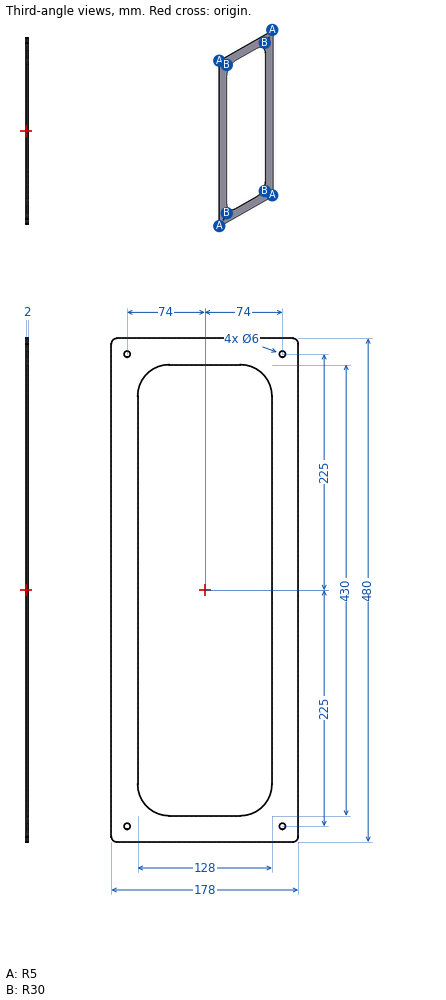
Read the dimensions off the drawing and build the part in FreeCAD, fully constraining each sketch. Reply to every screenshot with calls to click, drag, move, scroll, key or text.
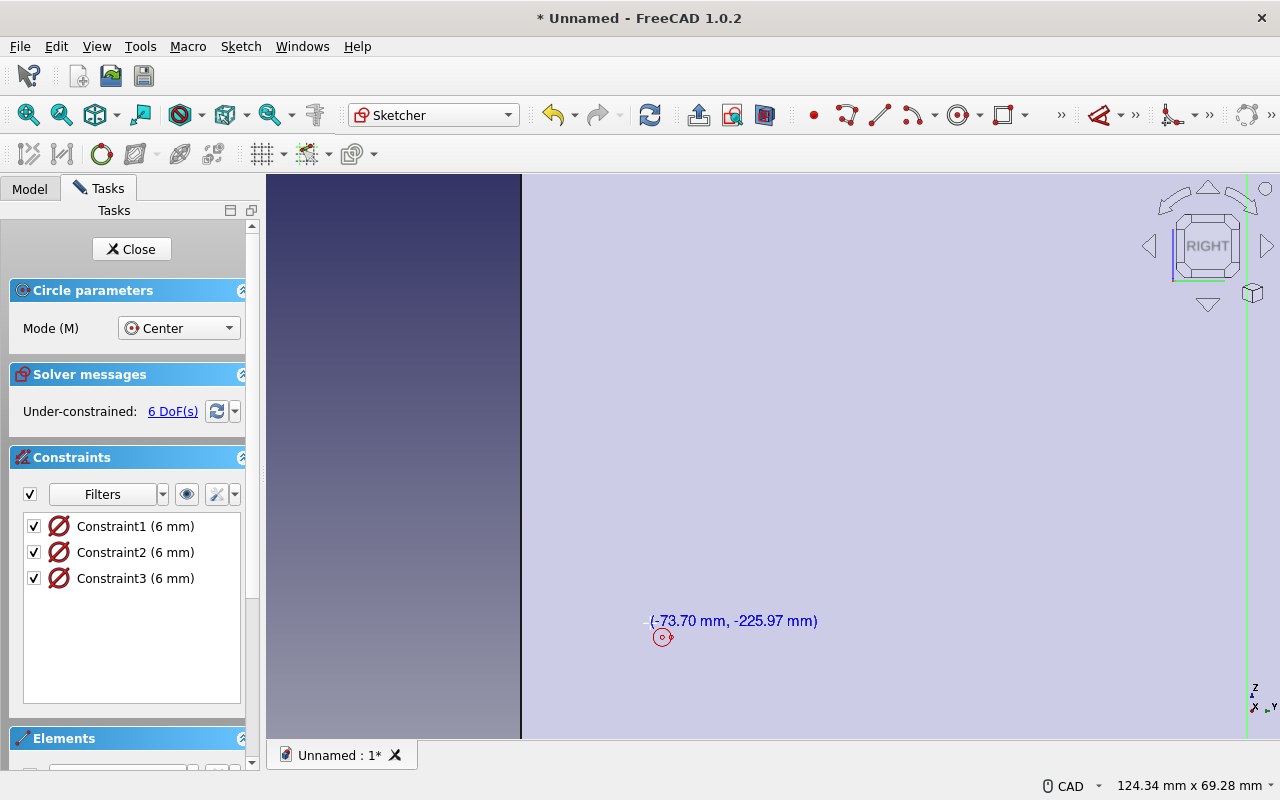
scroll(650, 623, down, 12)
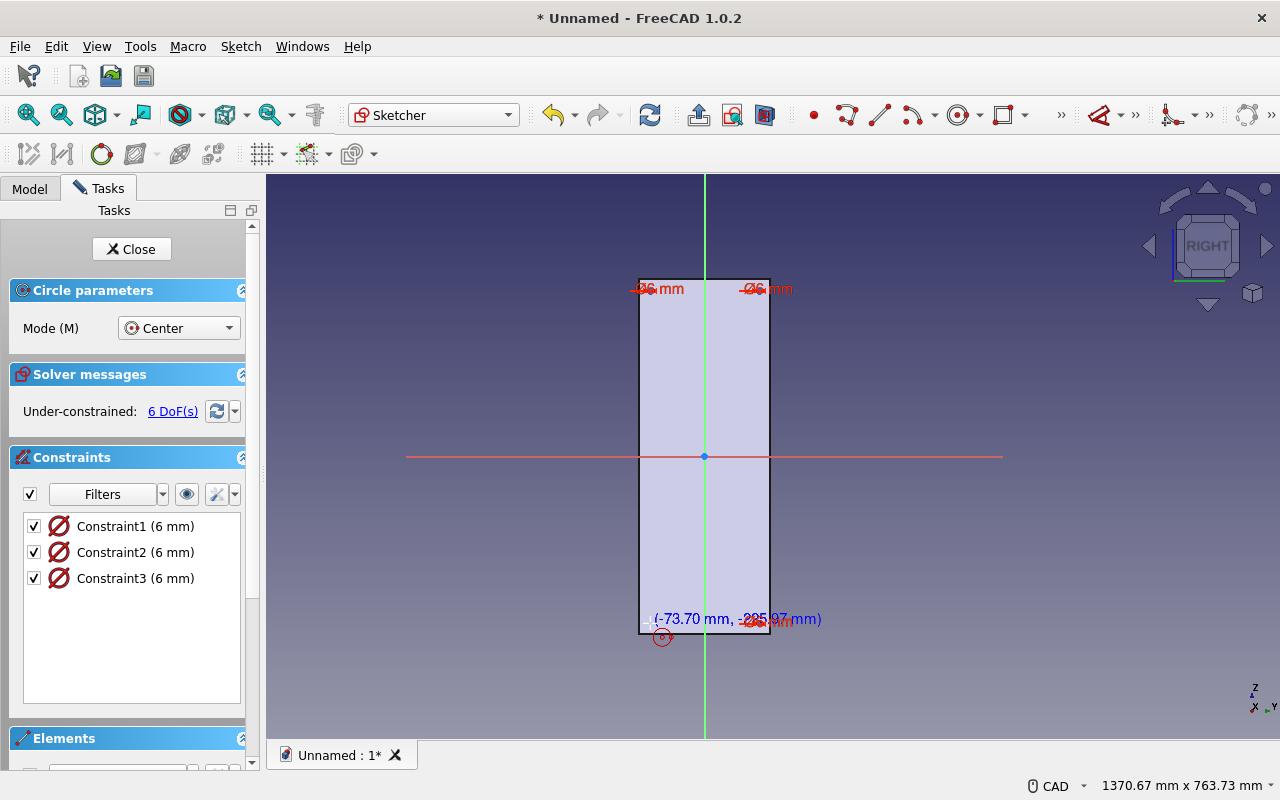
click(650, 623)
move(651, 622)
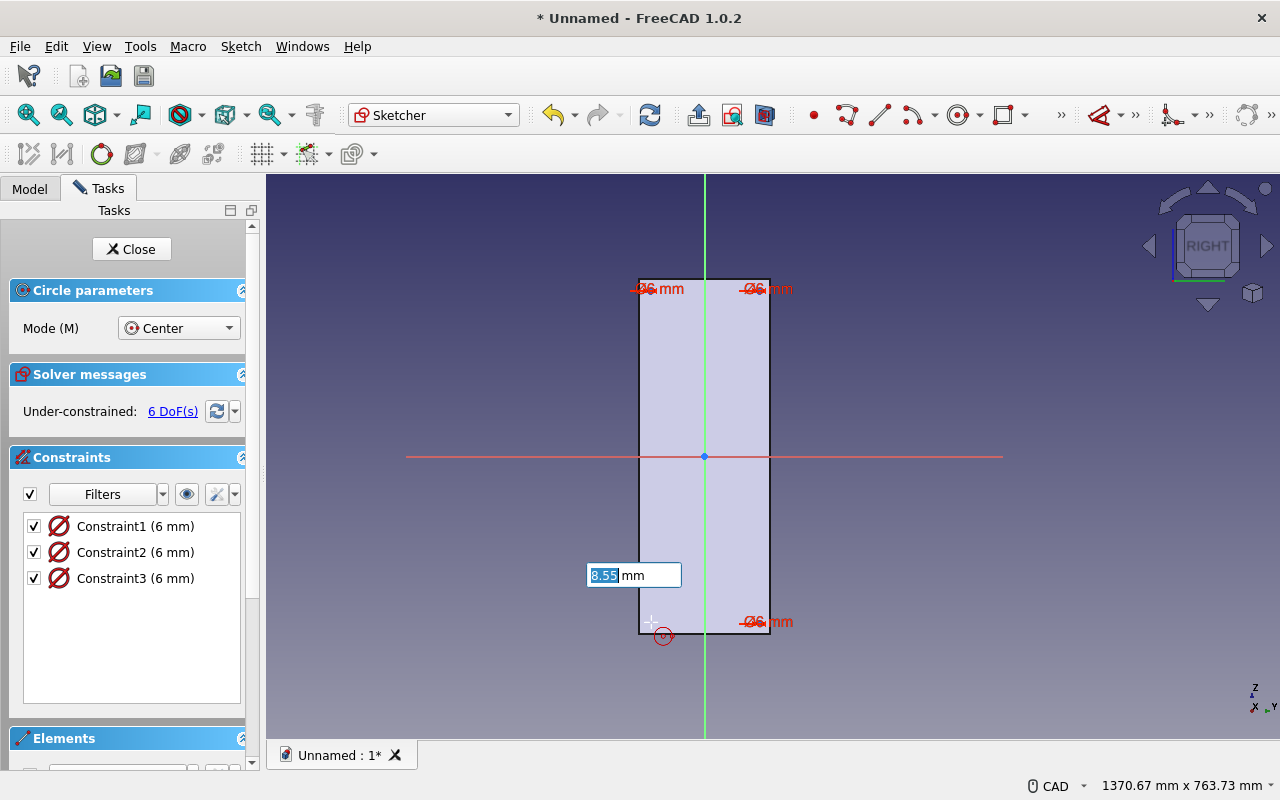
text(6)
key(Return)
key(Escape)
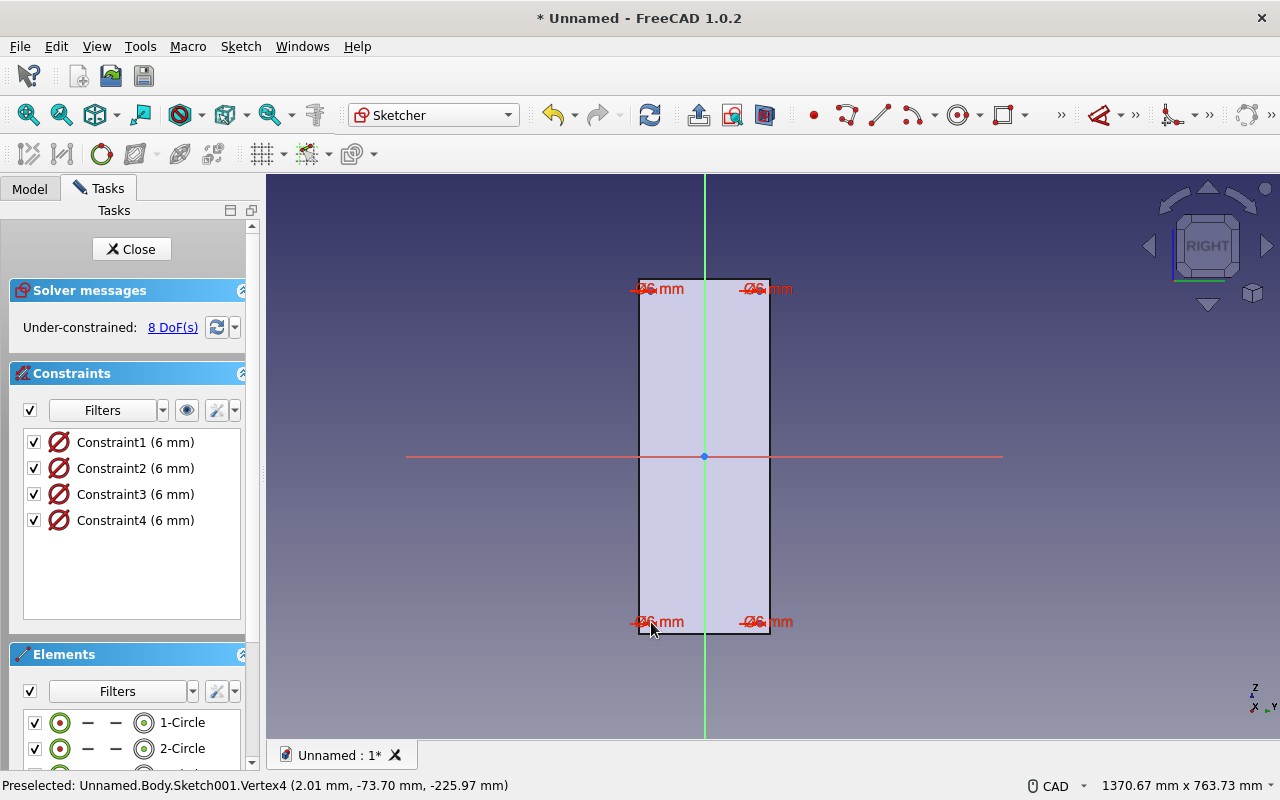
click(759, 291)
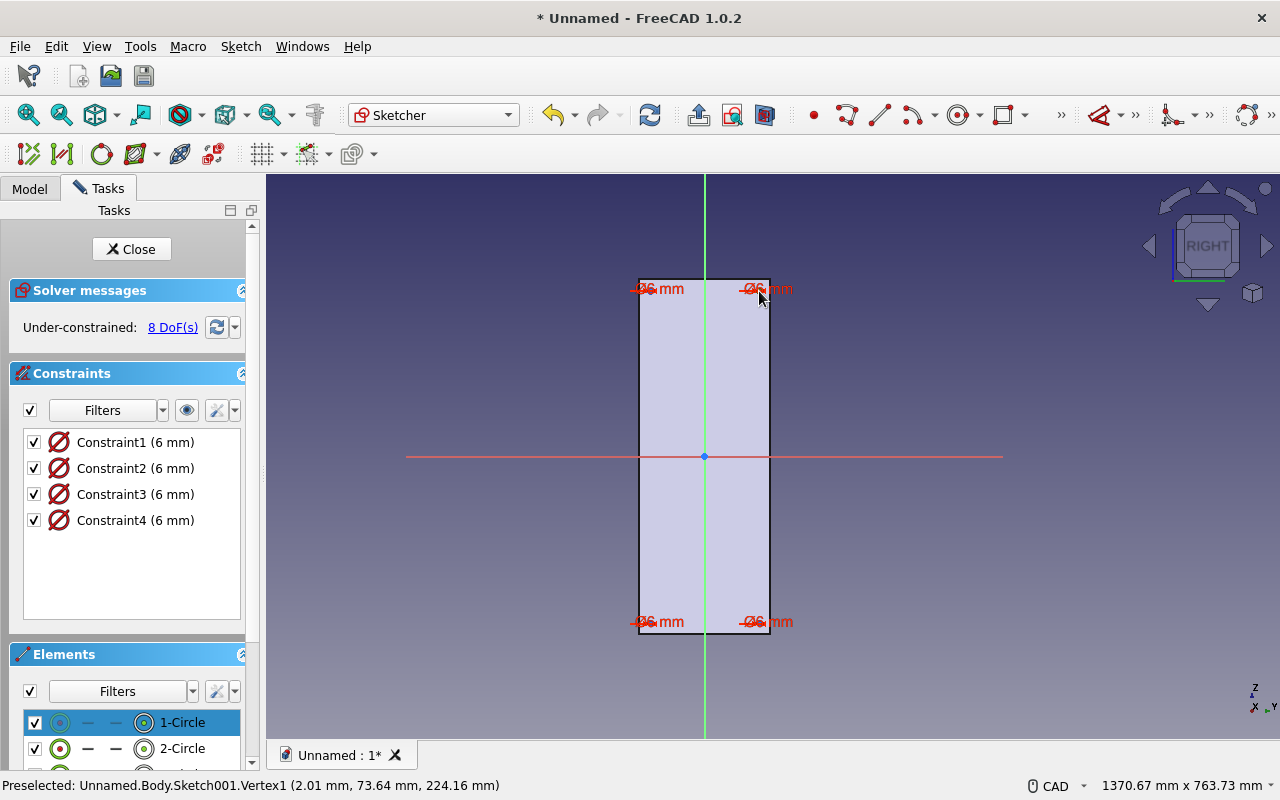
click(759, 624)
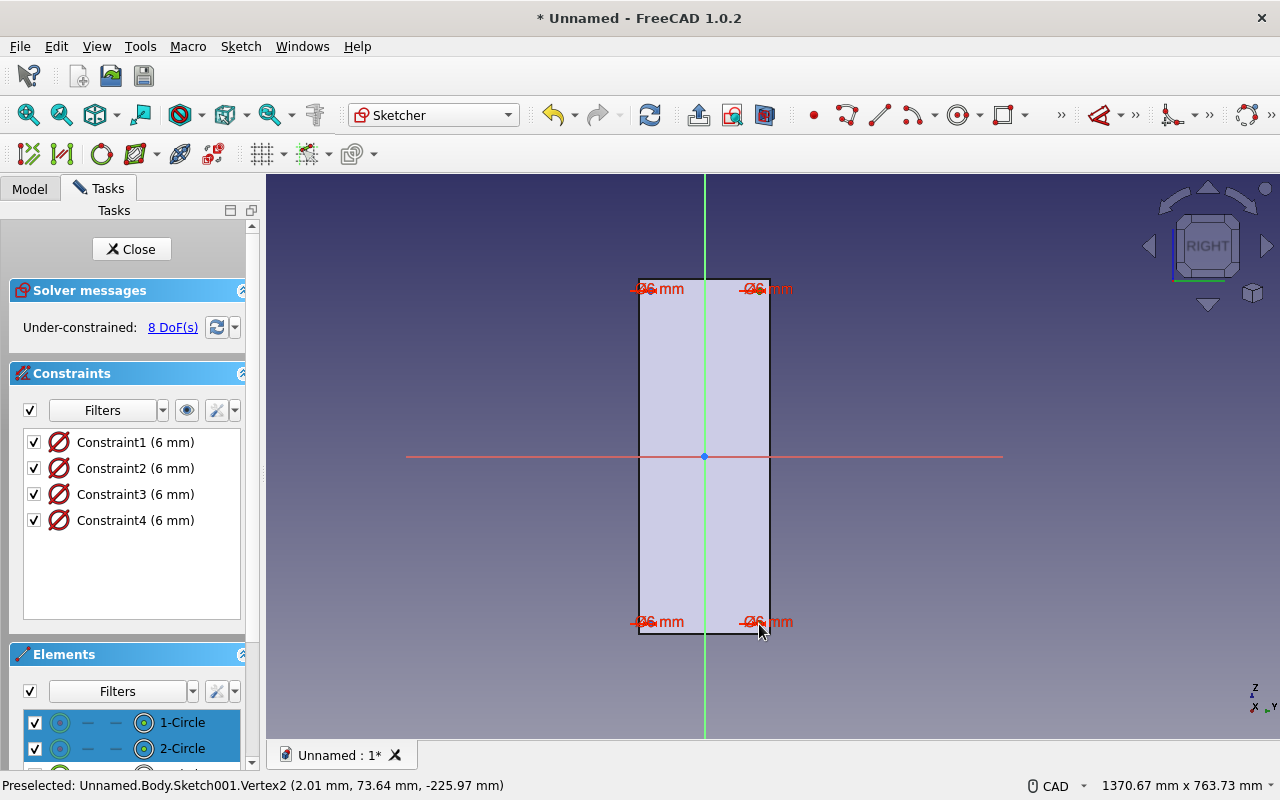
key(v)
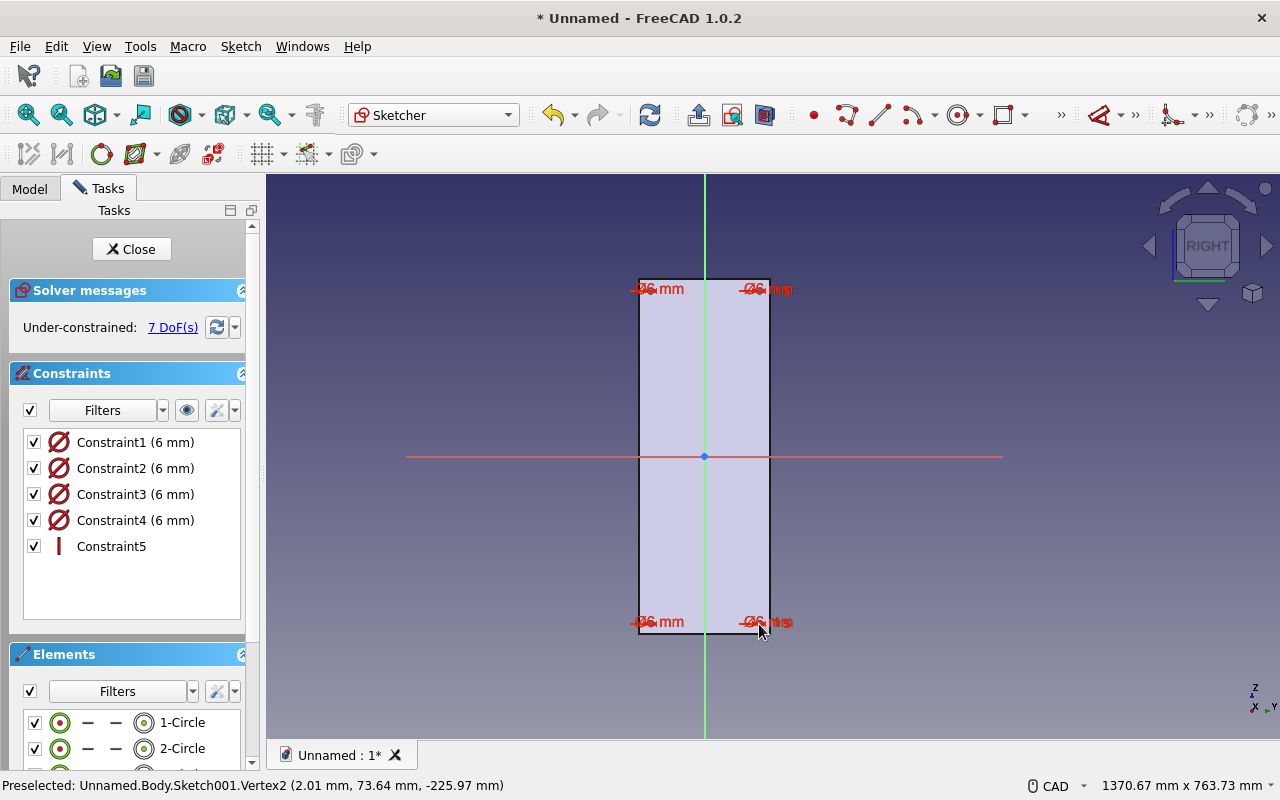
click(759, 291)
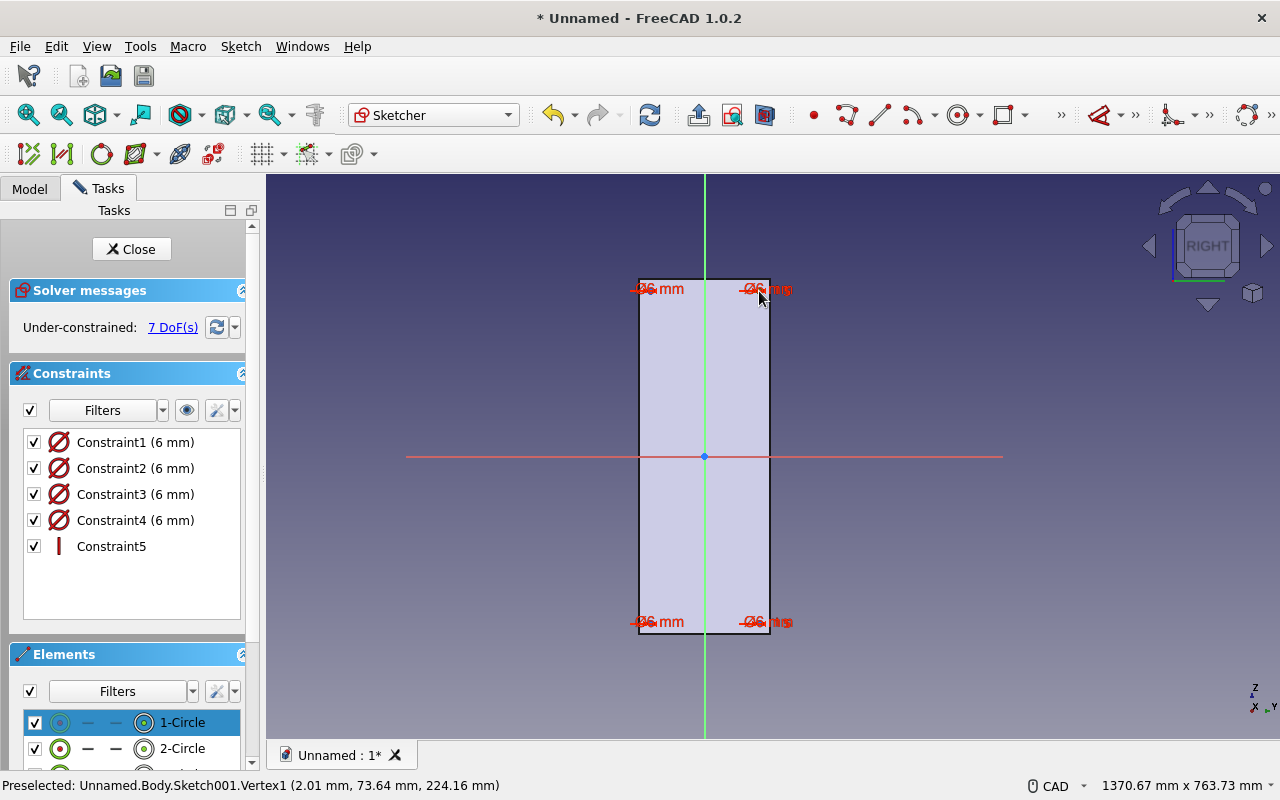
click(650, 291)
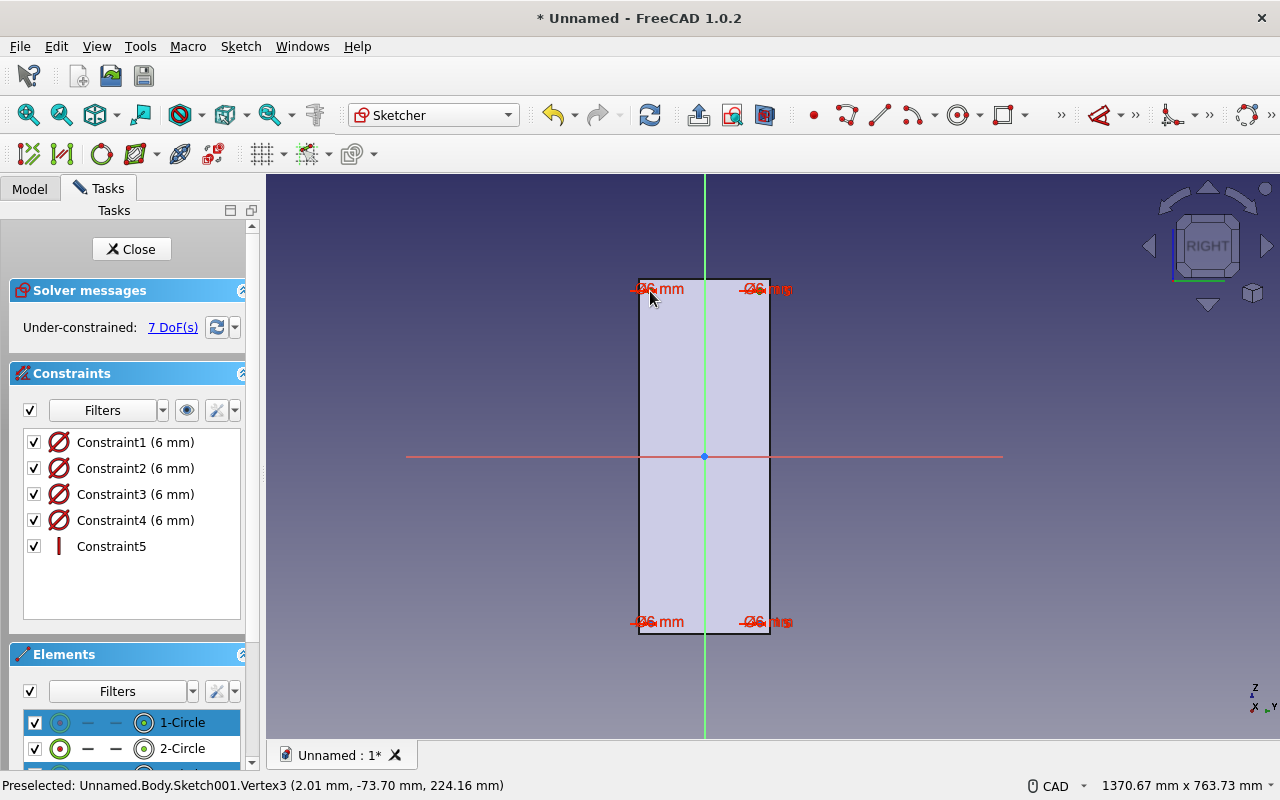
key(h)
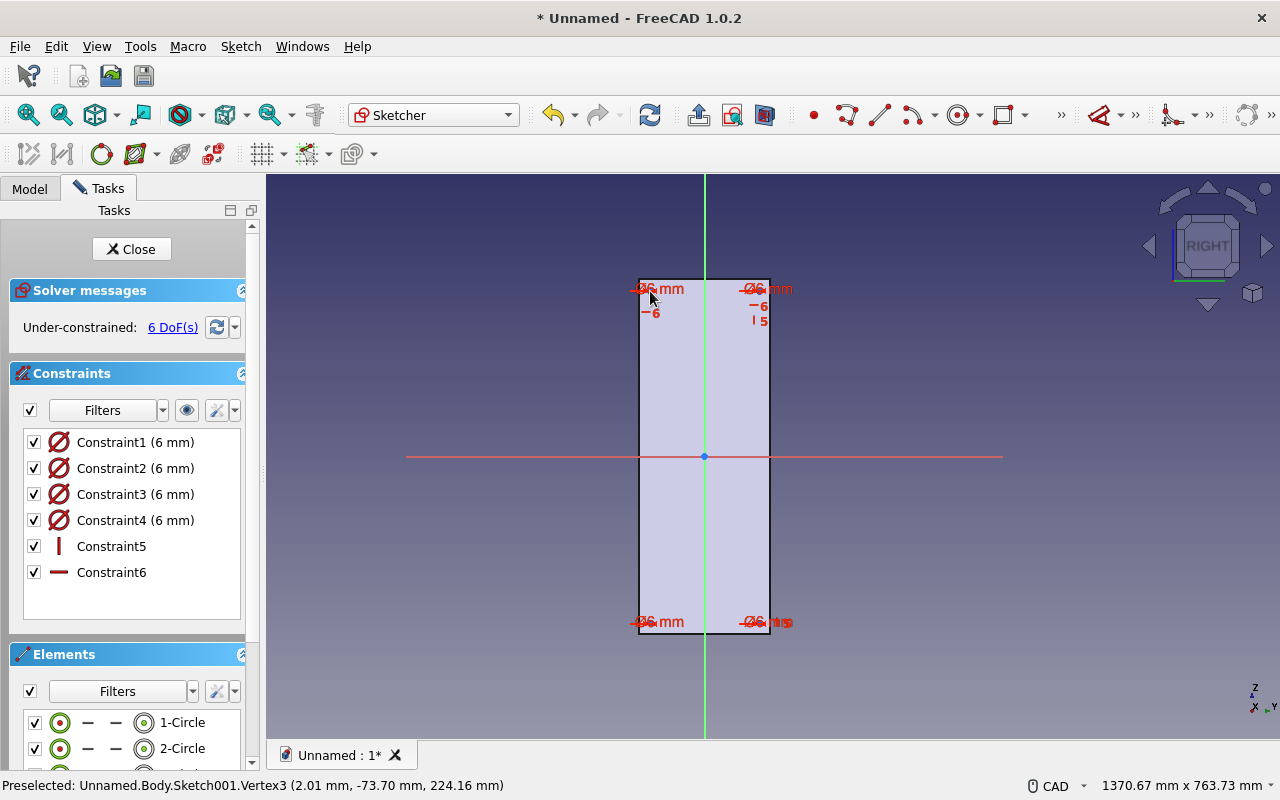
click(650, 291)